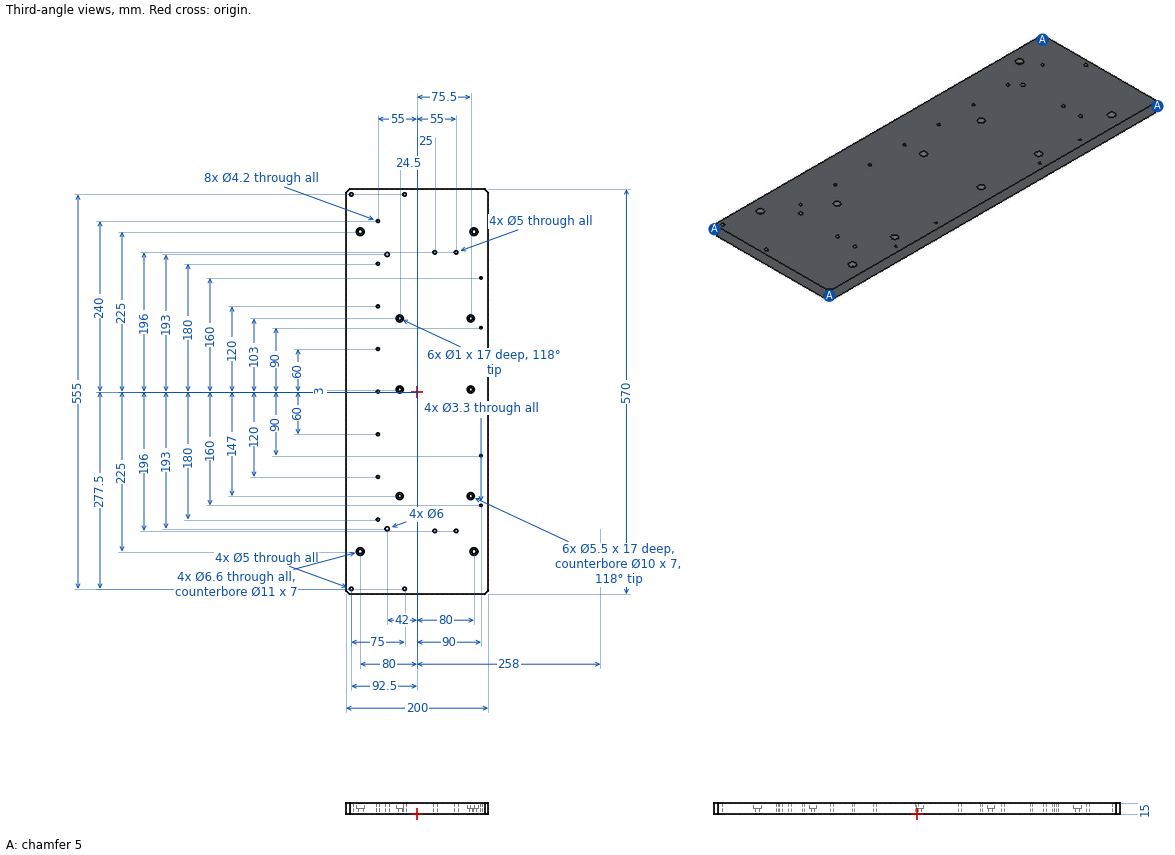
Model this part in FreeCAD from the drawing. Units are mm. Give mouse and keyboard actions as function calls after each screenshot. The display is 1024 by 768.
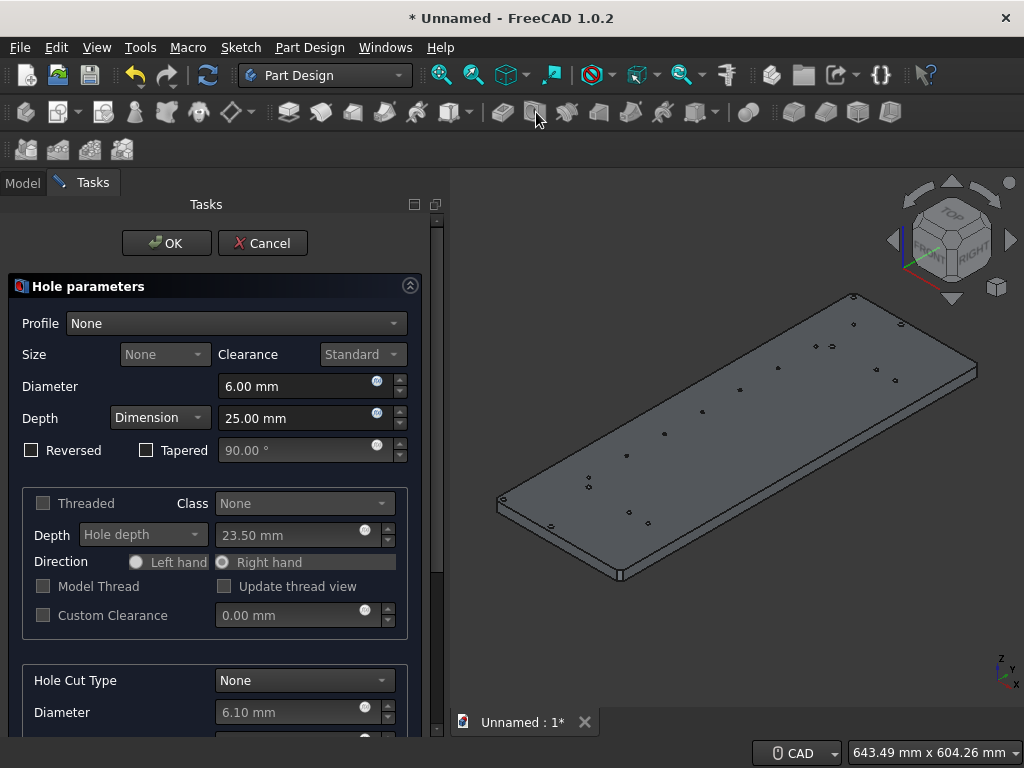
triple_click(305, 386)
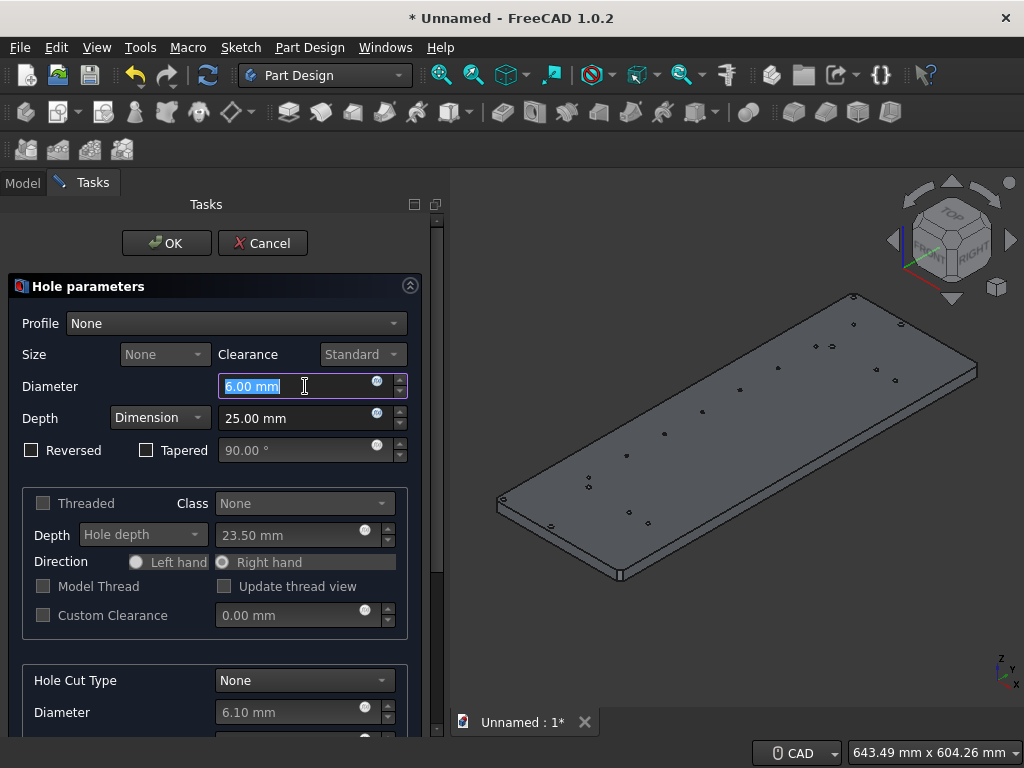
text(5)
key(Tab)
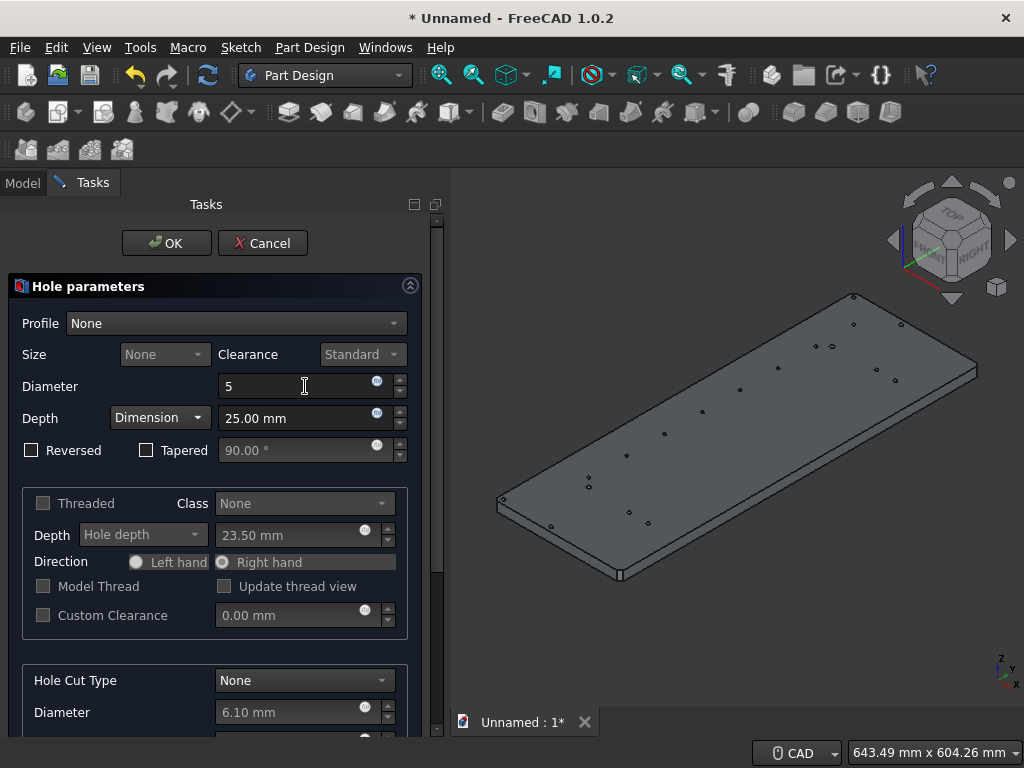
click(161, 418)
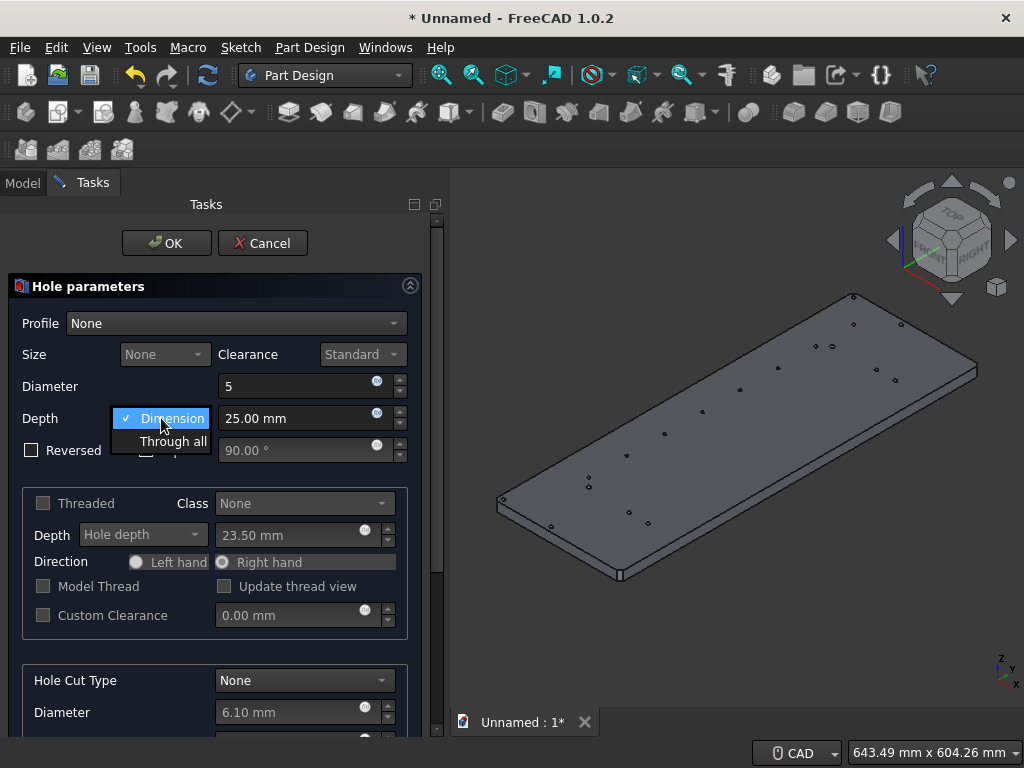
click(160, 442)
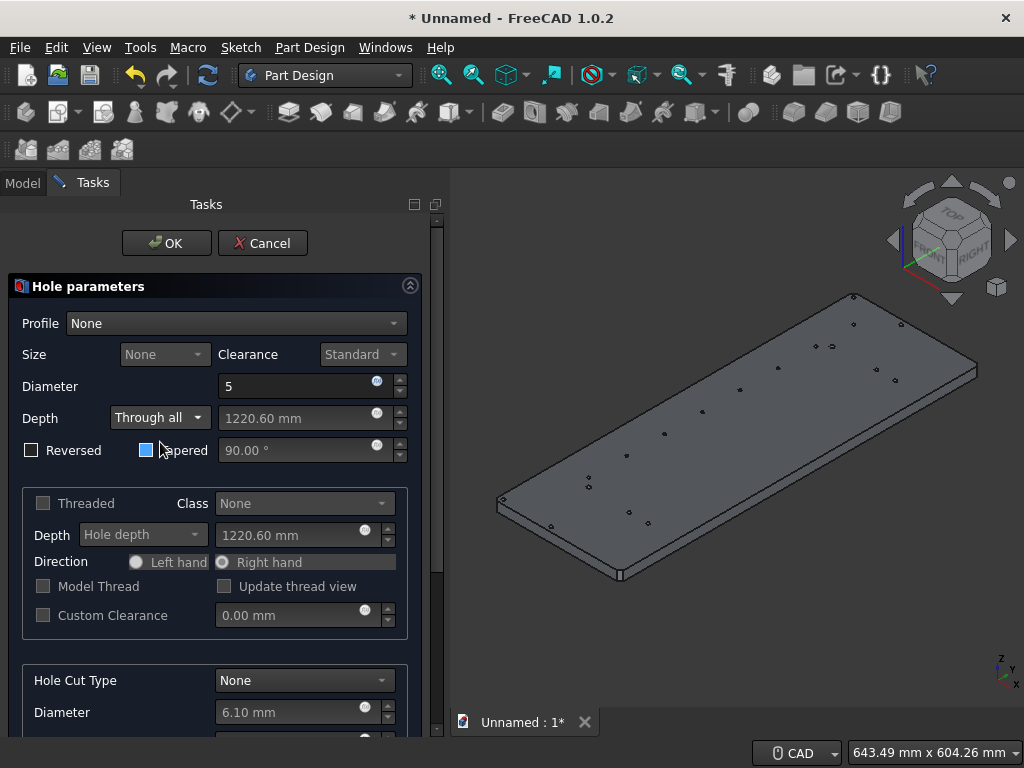
click(167, 243)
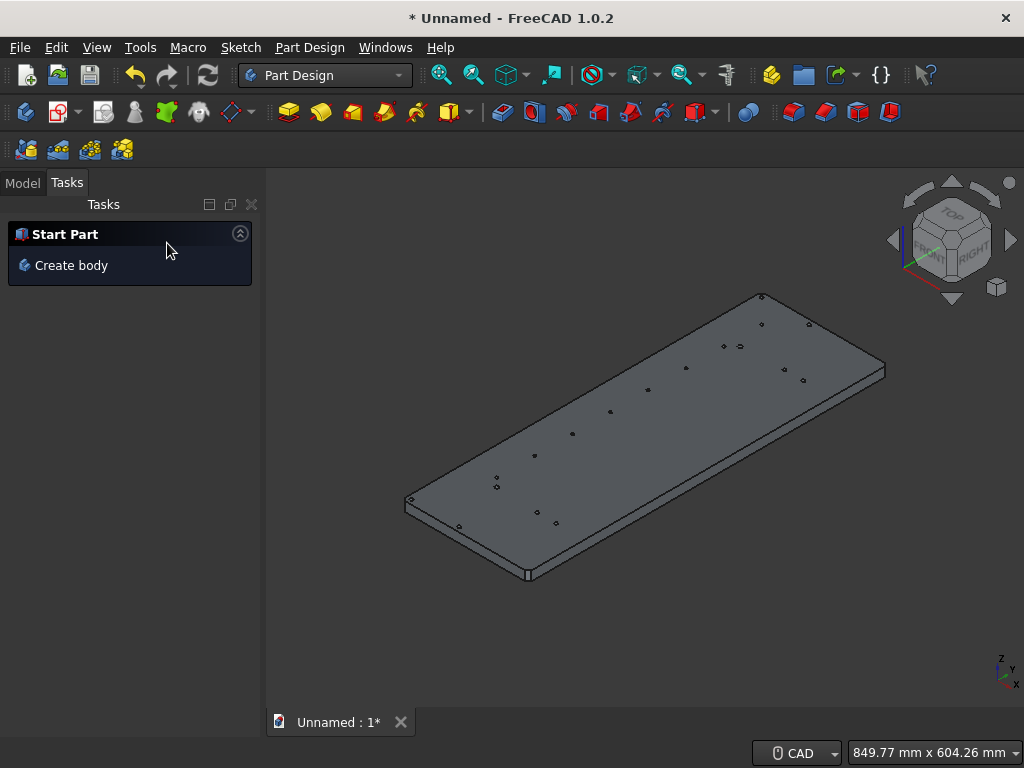
click(714, 412)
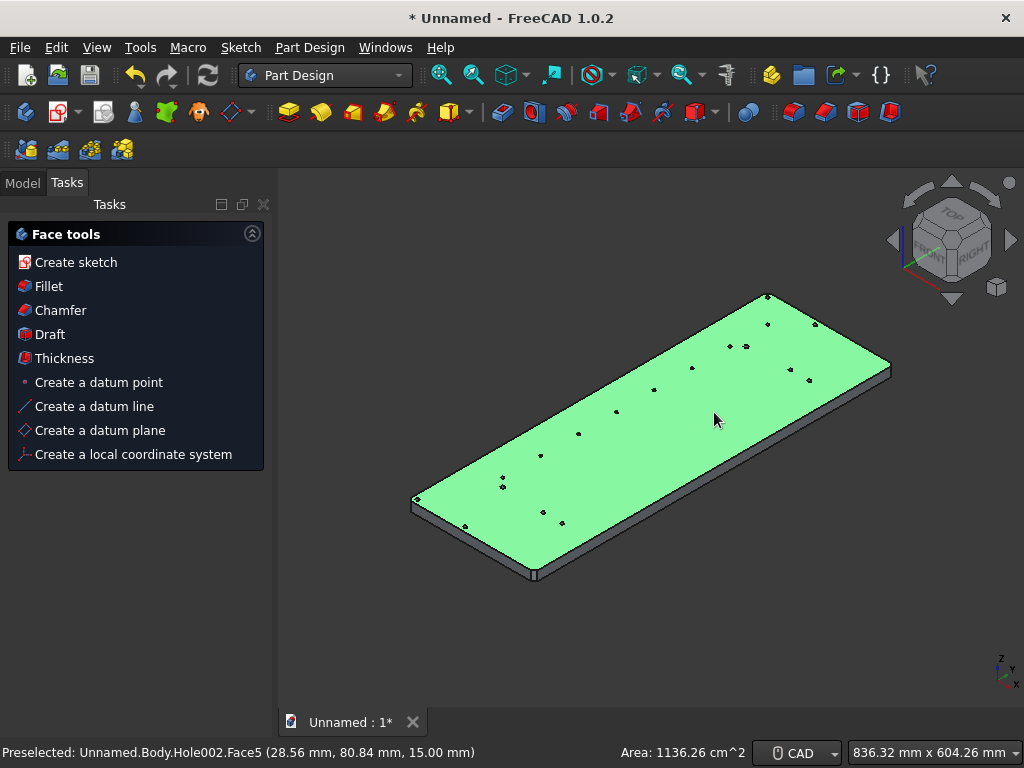
click(58, 112)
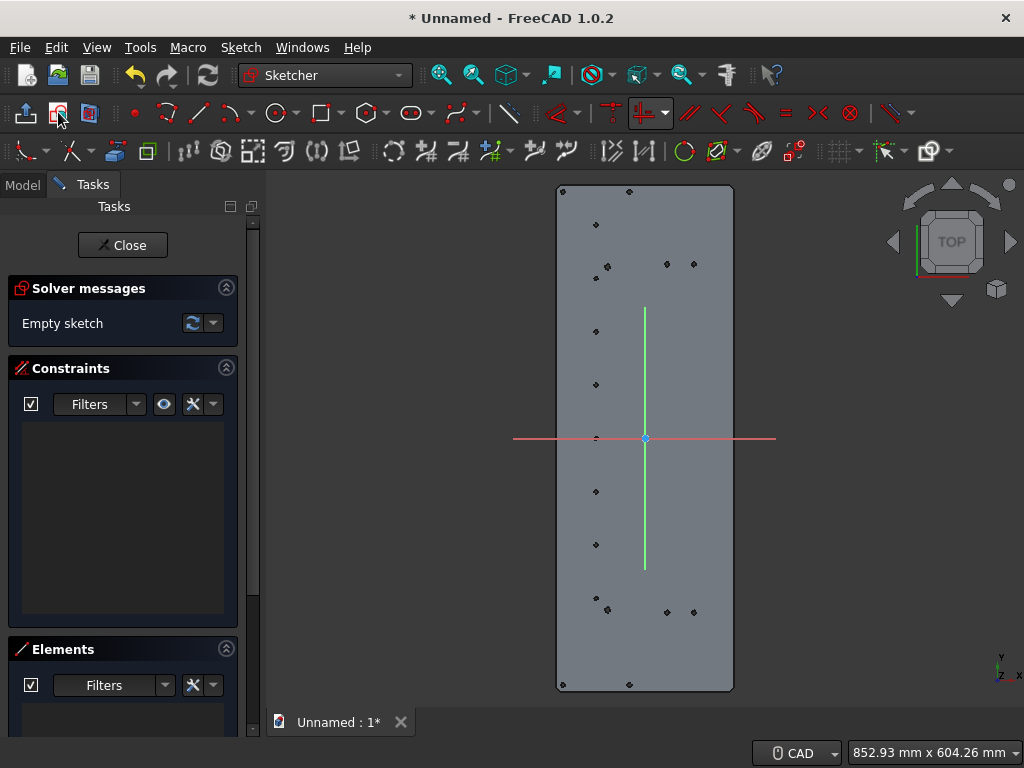
click(276, 114)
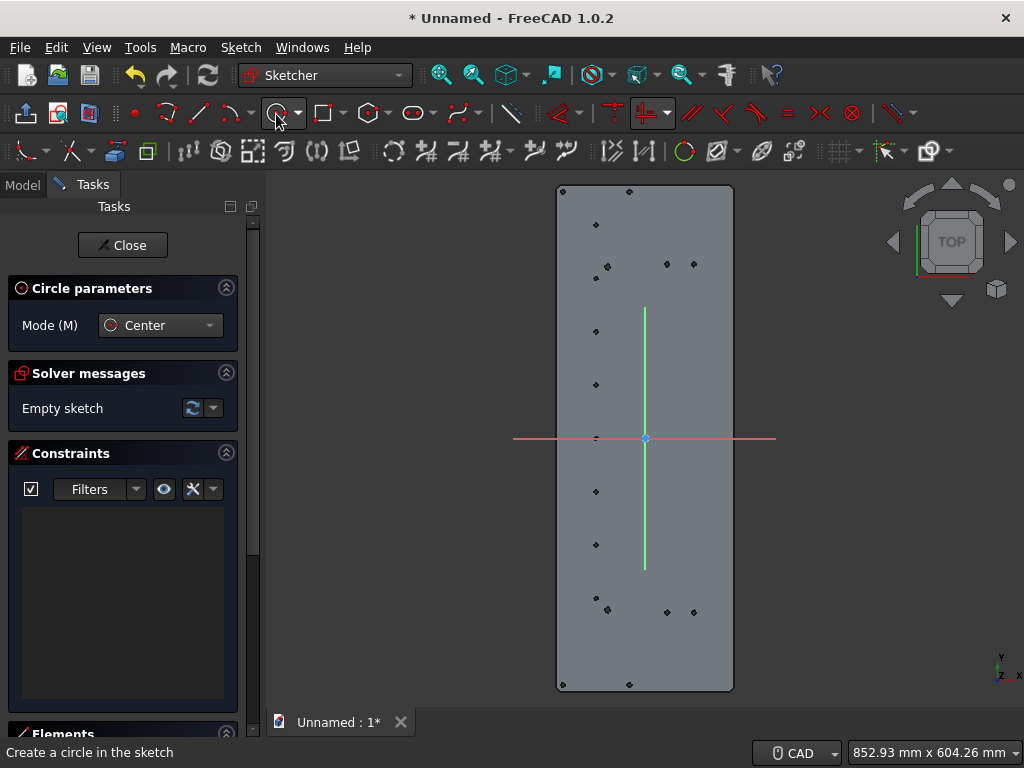
scroll(725, 581, up, 14)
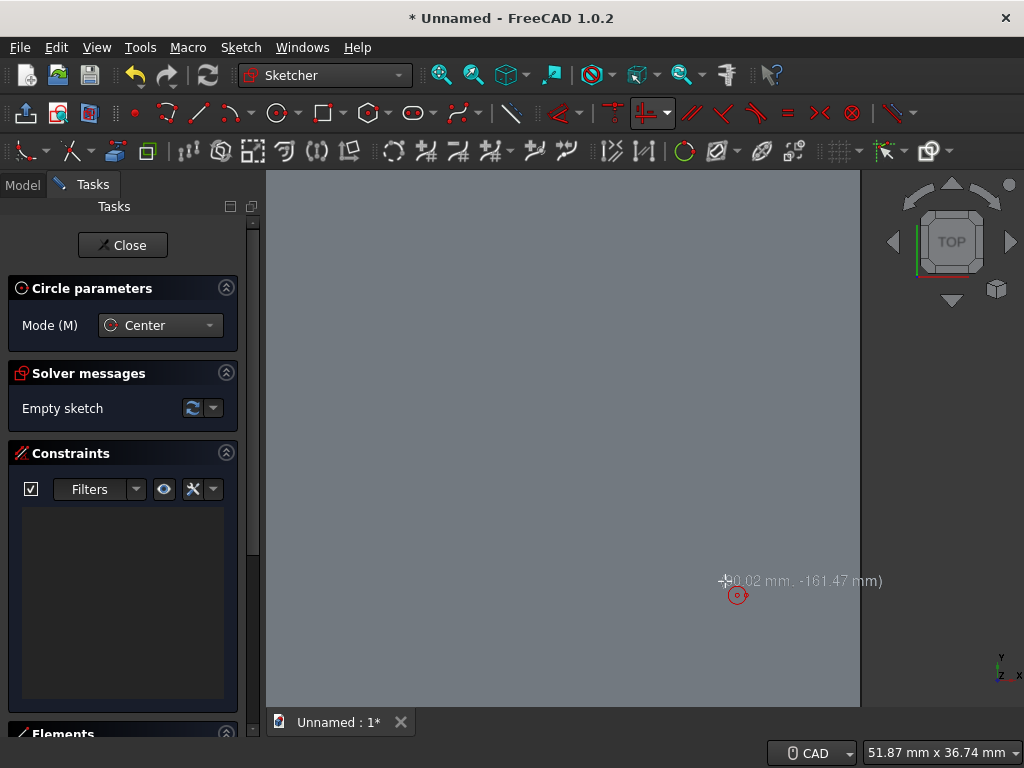
scroll(617, 616, down, 13)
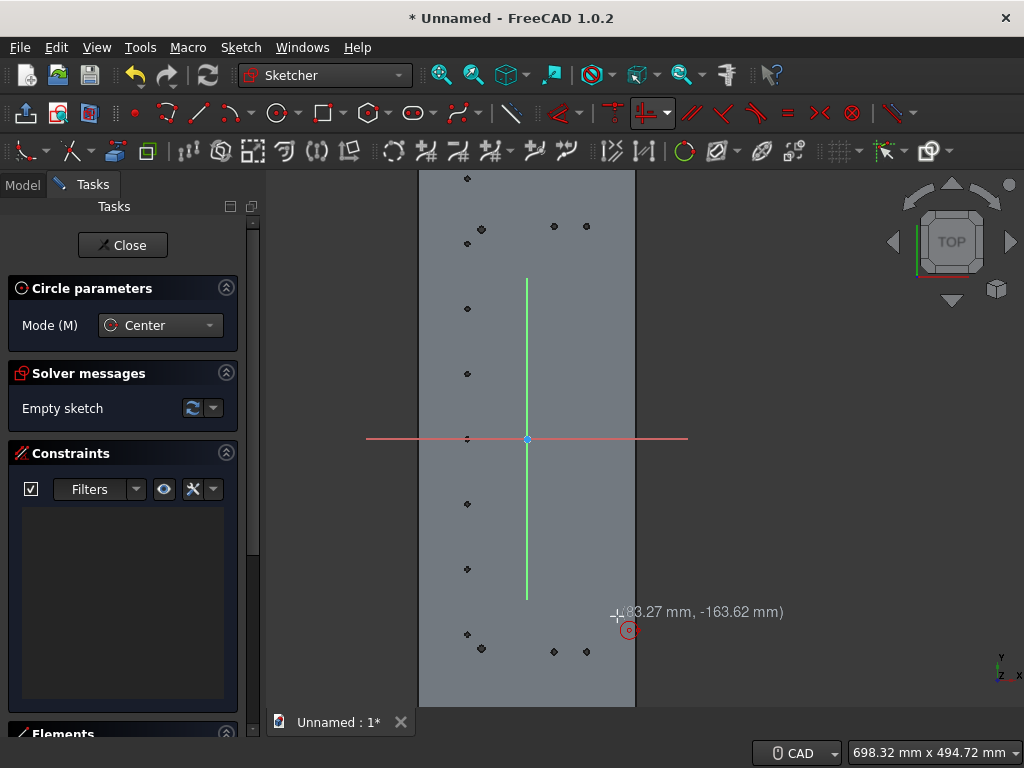
click(625, 613)
move(626, 612)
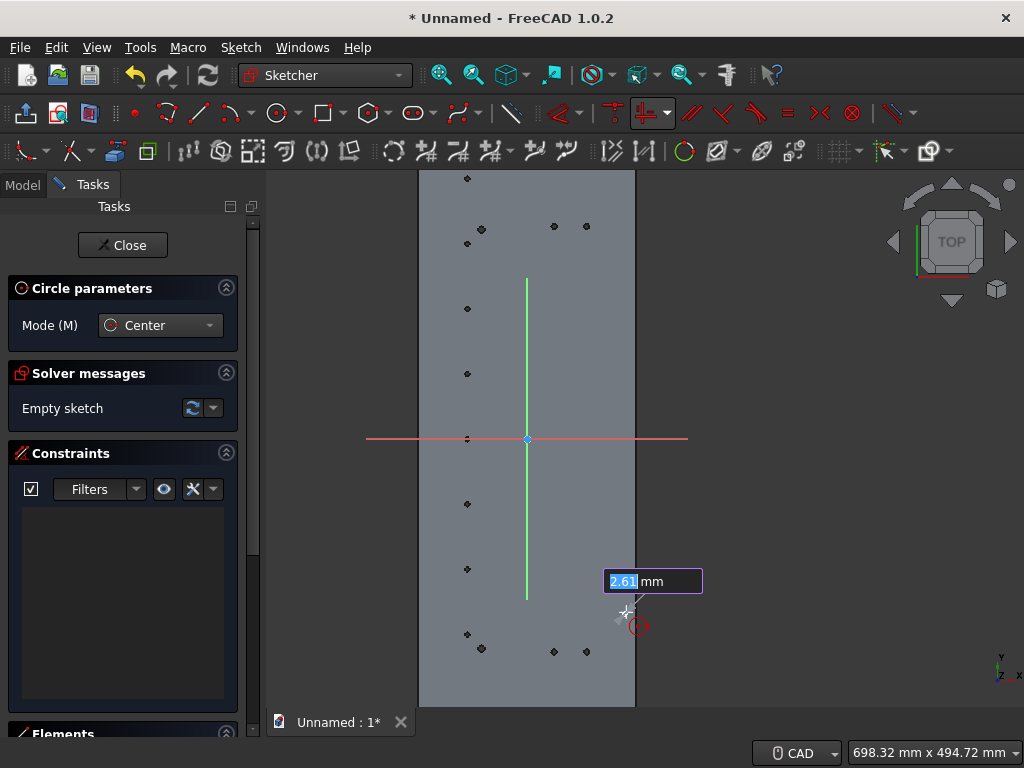
text(3.3)
key(Return)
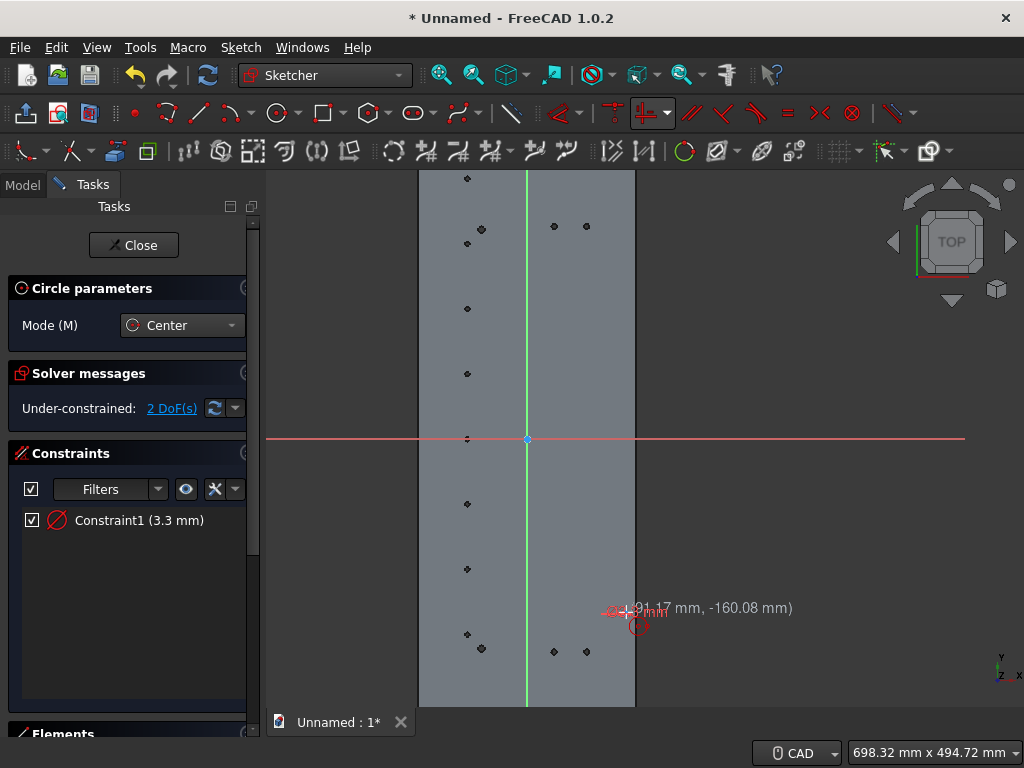
scroll(625, 537, up, 13)